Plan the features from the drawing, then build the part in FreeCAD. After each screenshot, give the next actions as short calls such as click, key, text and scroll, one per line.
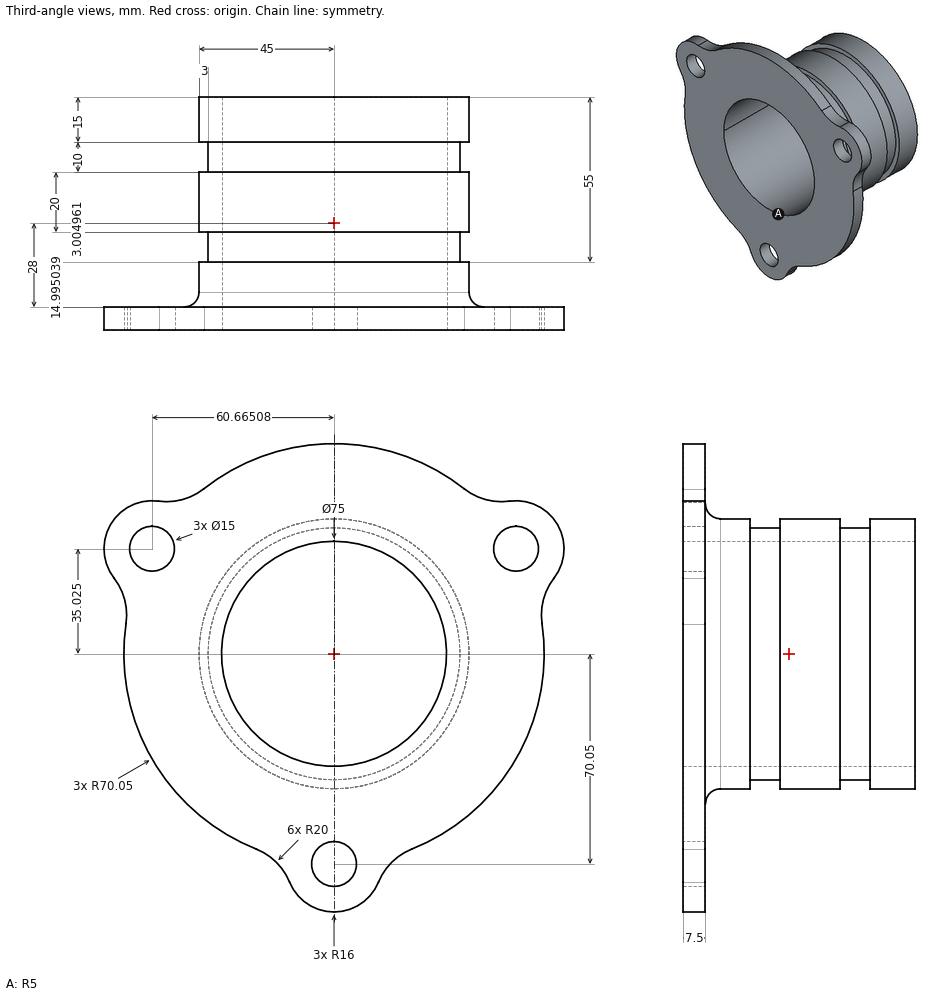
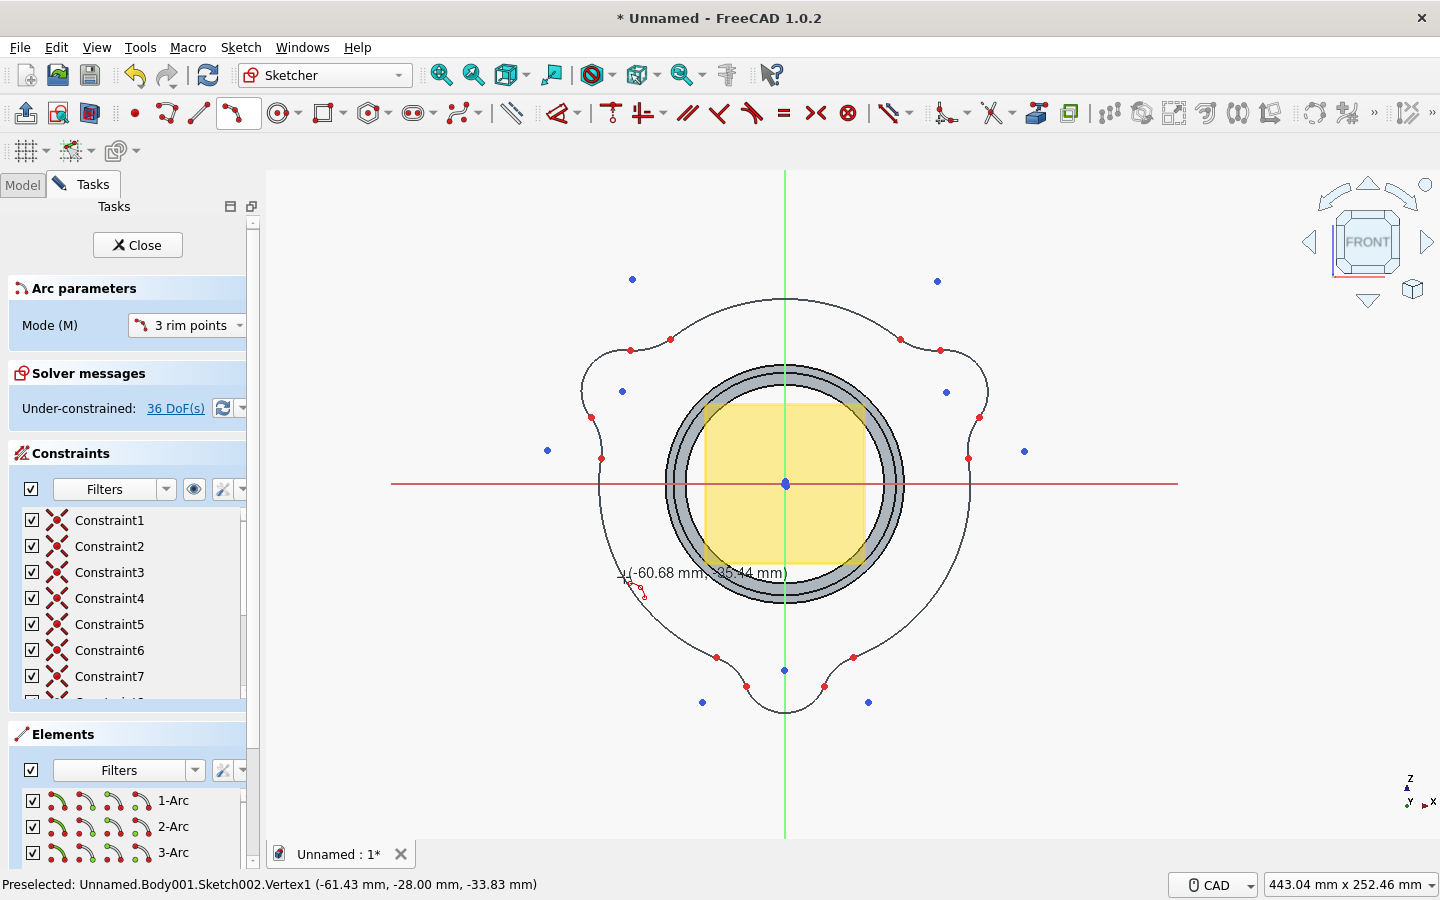
key(g)
key(c)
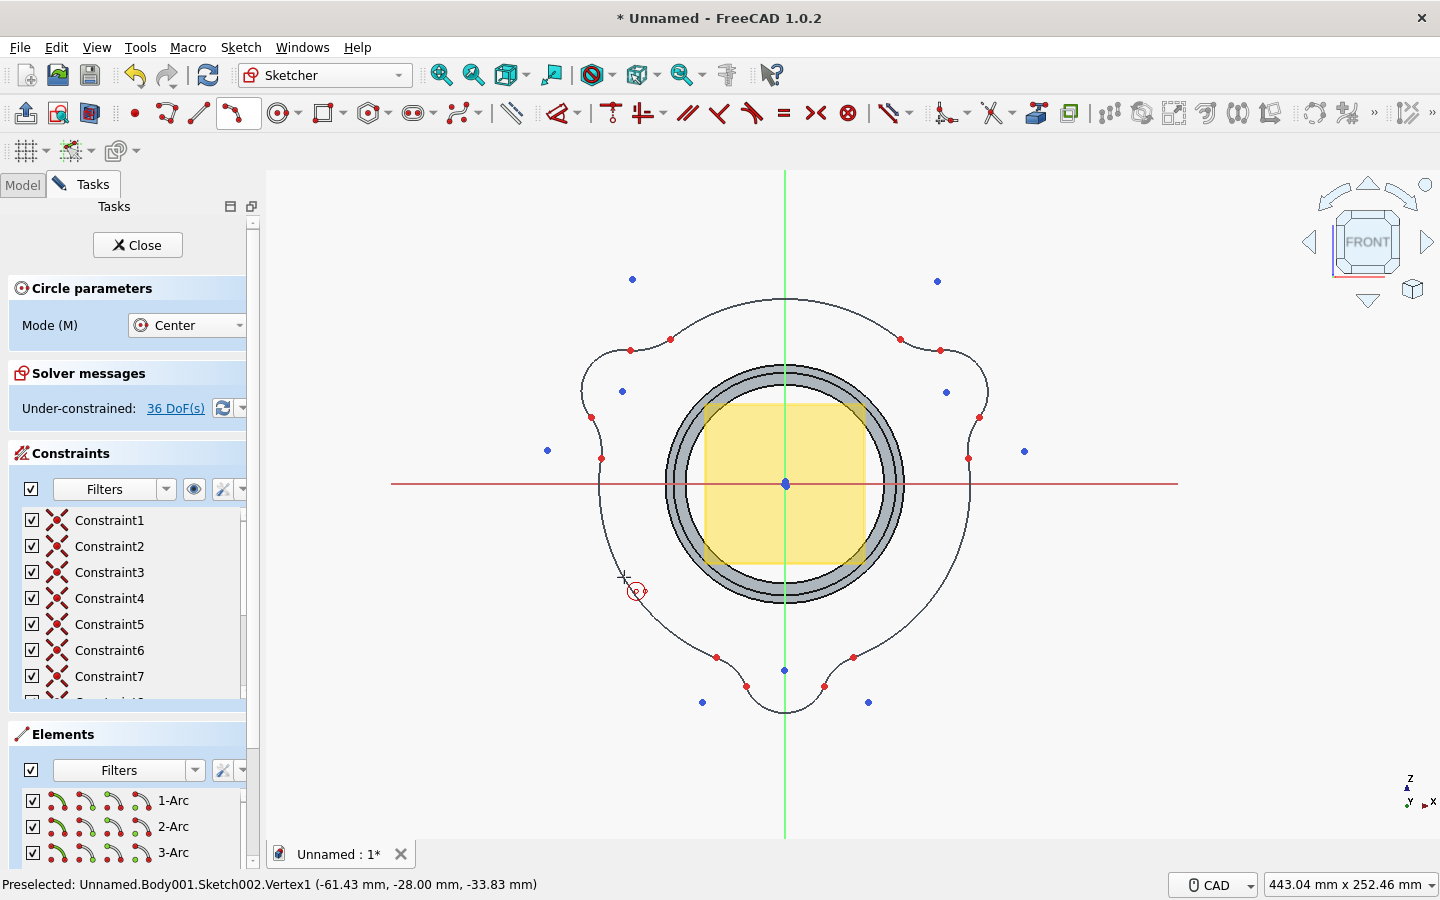
click(624, 391)
click(638, 377)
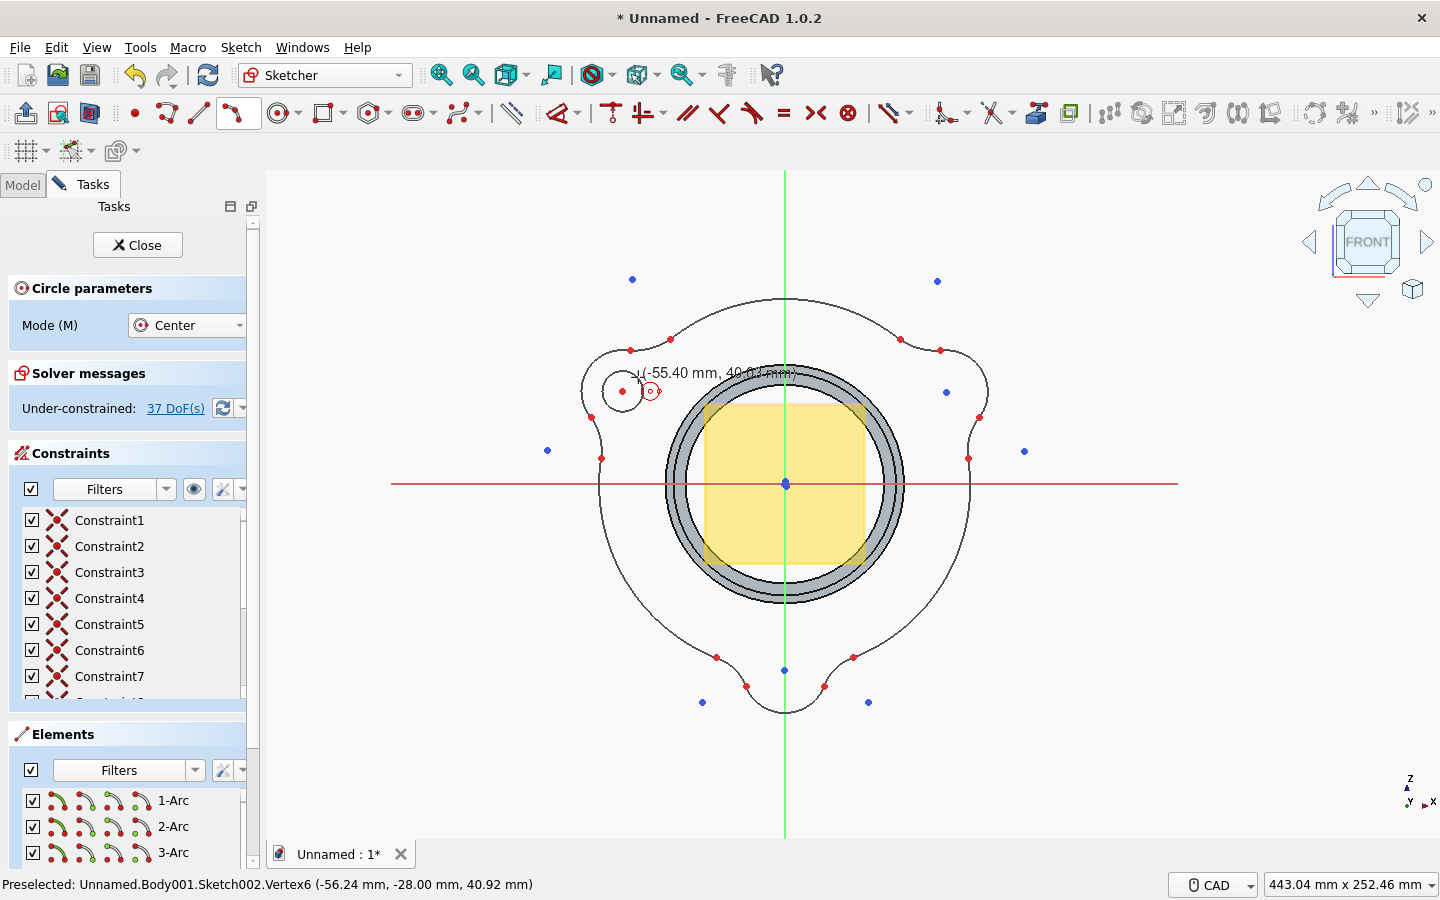
click(946, 391)
click(960, 377)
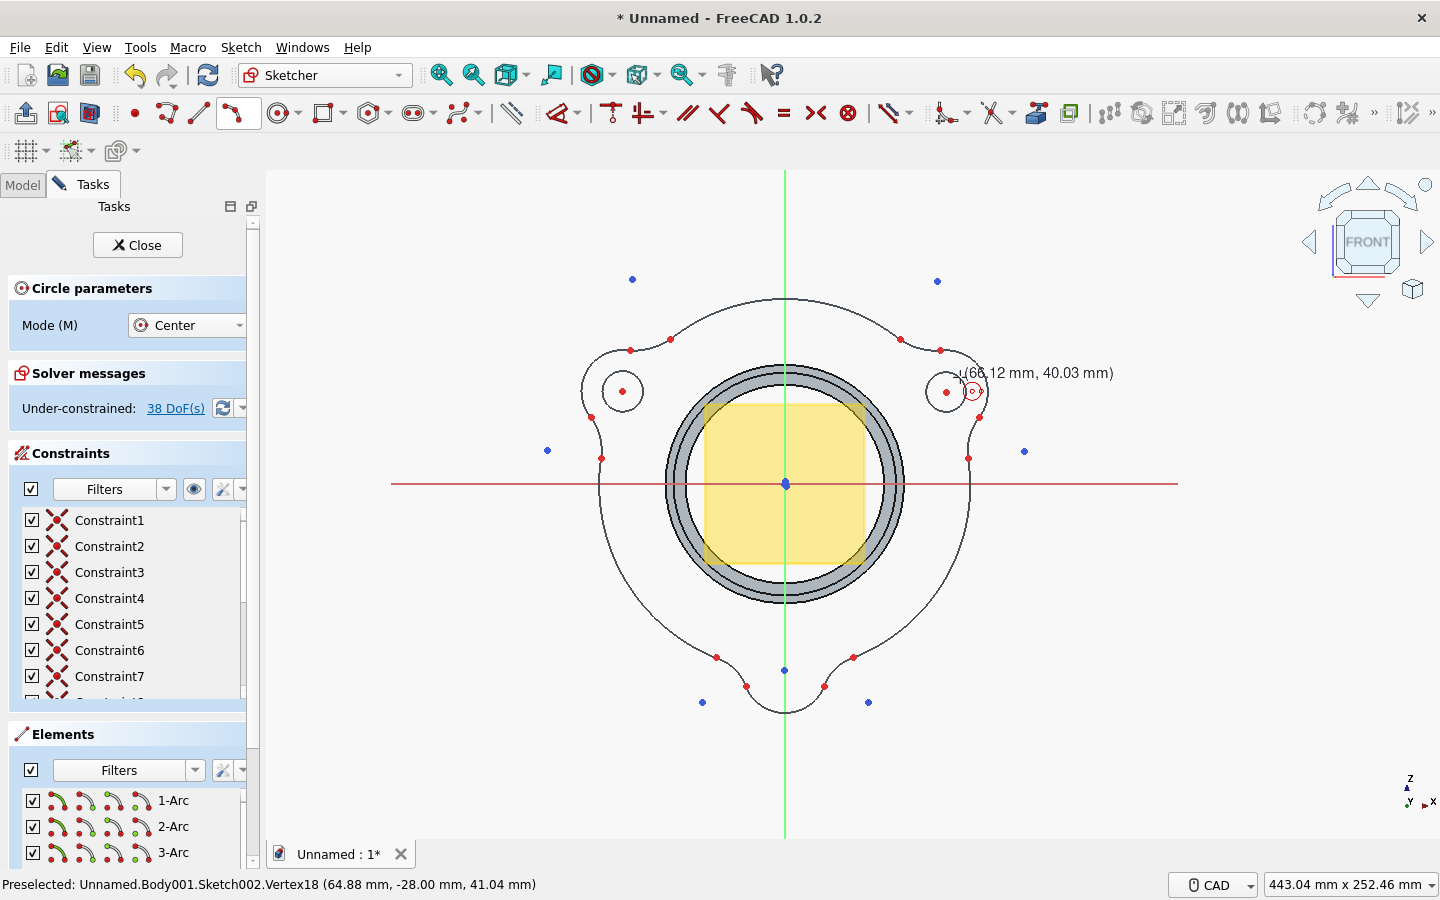
click(785, 670)
click(799, 656)
key(Escape)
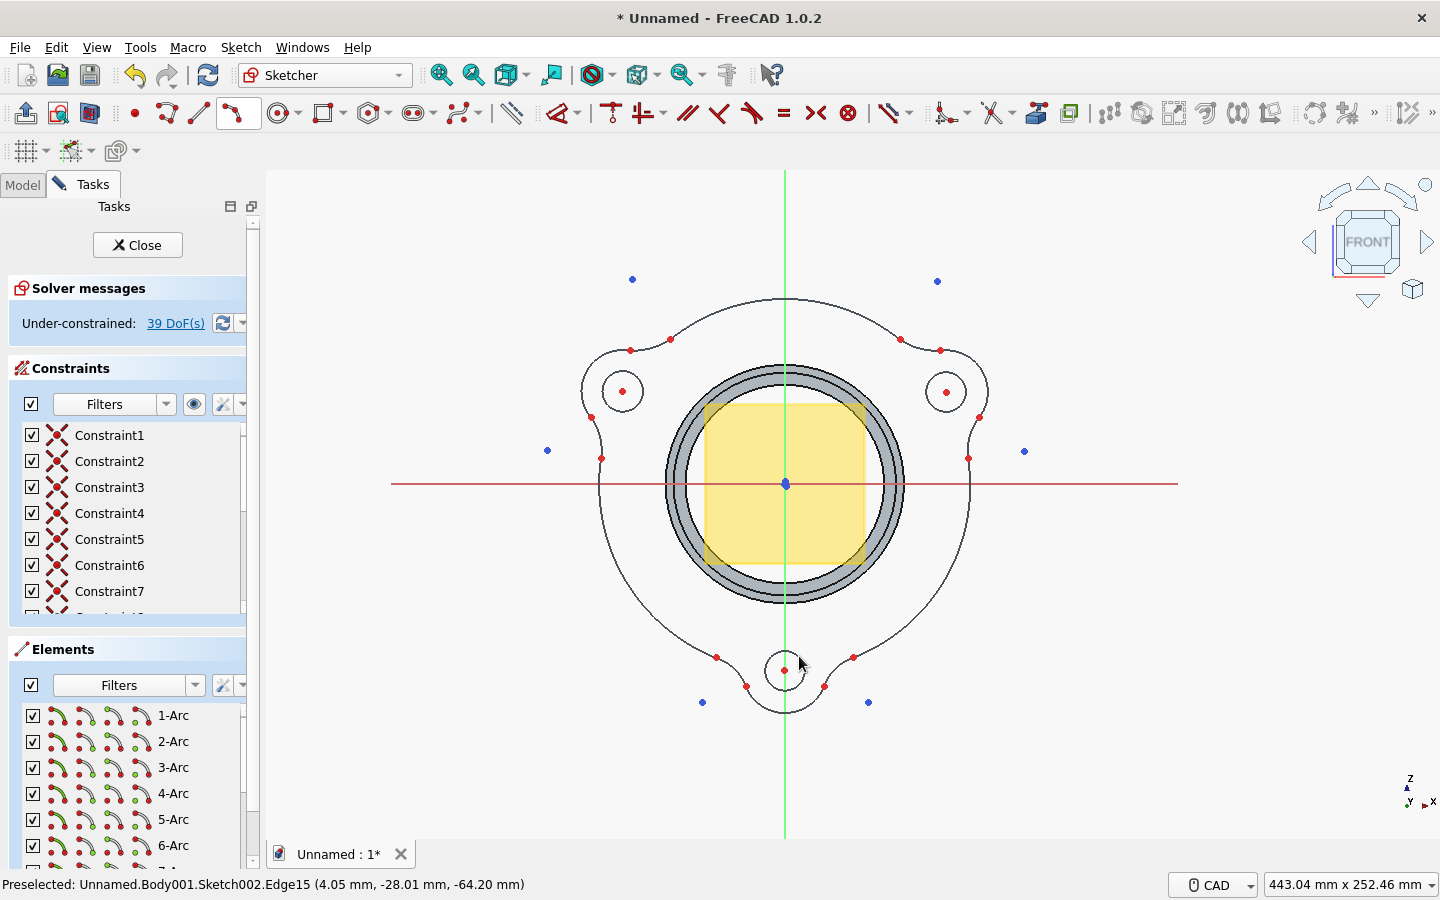
click(602, 446)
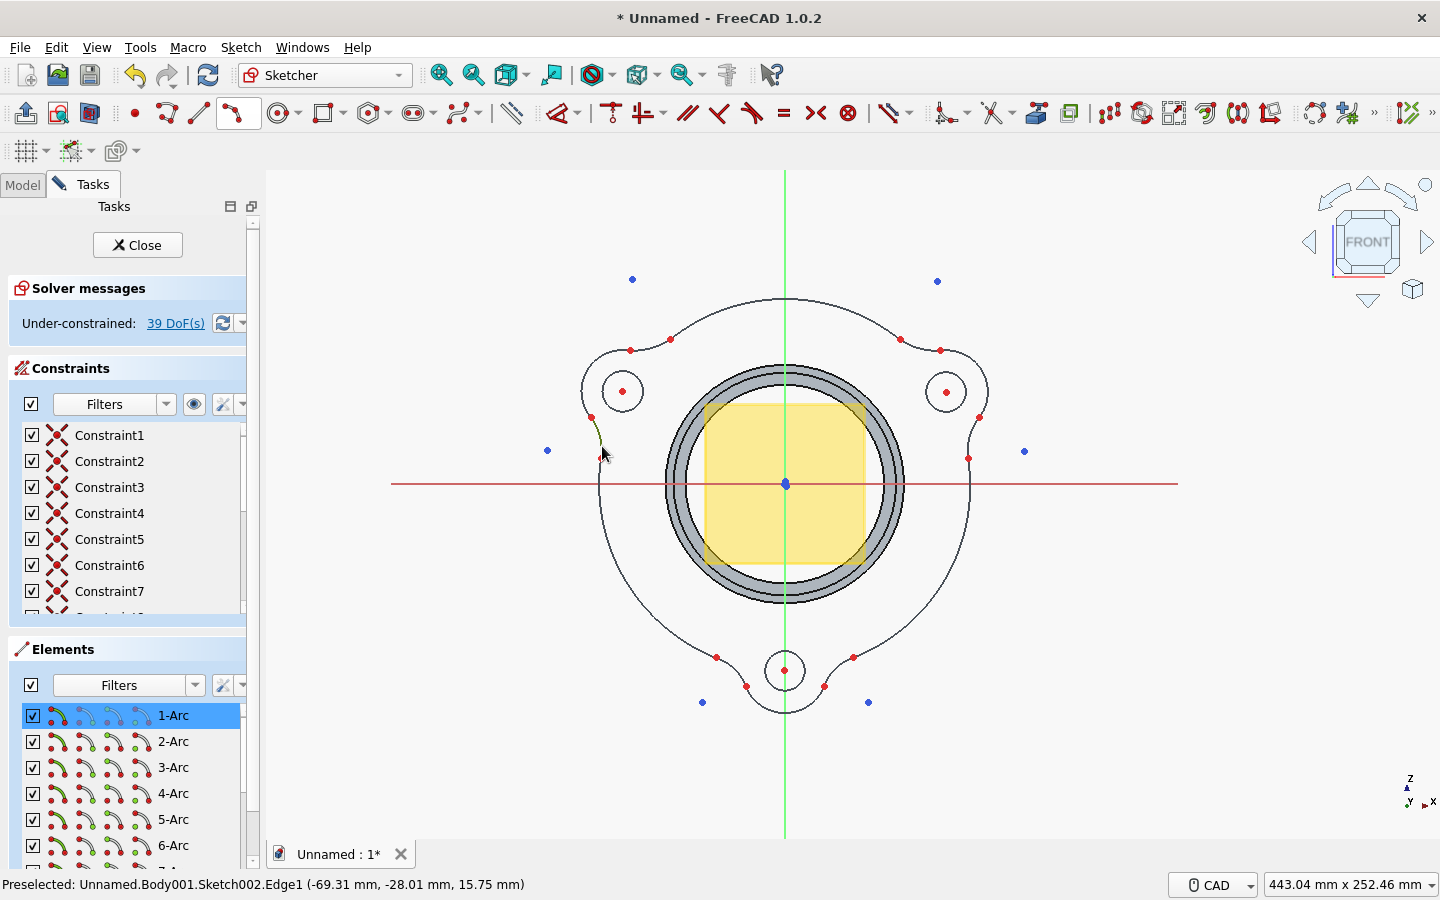
click(601, 356)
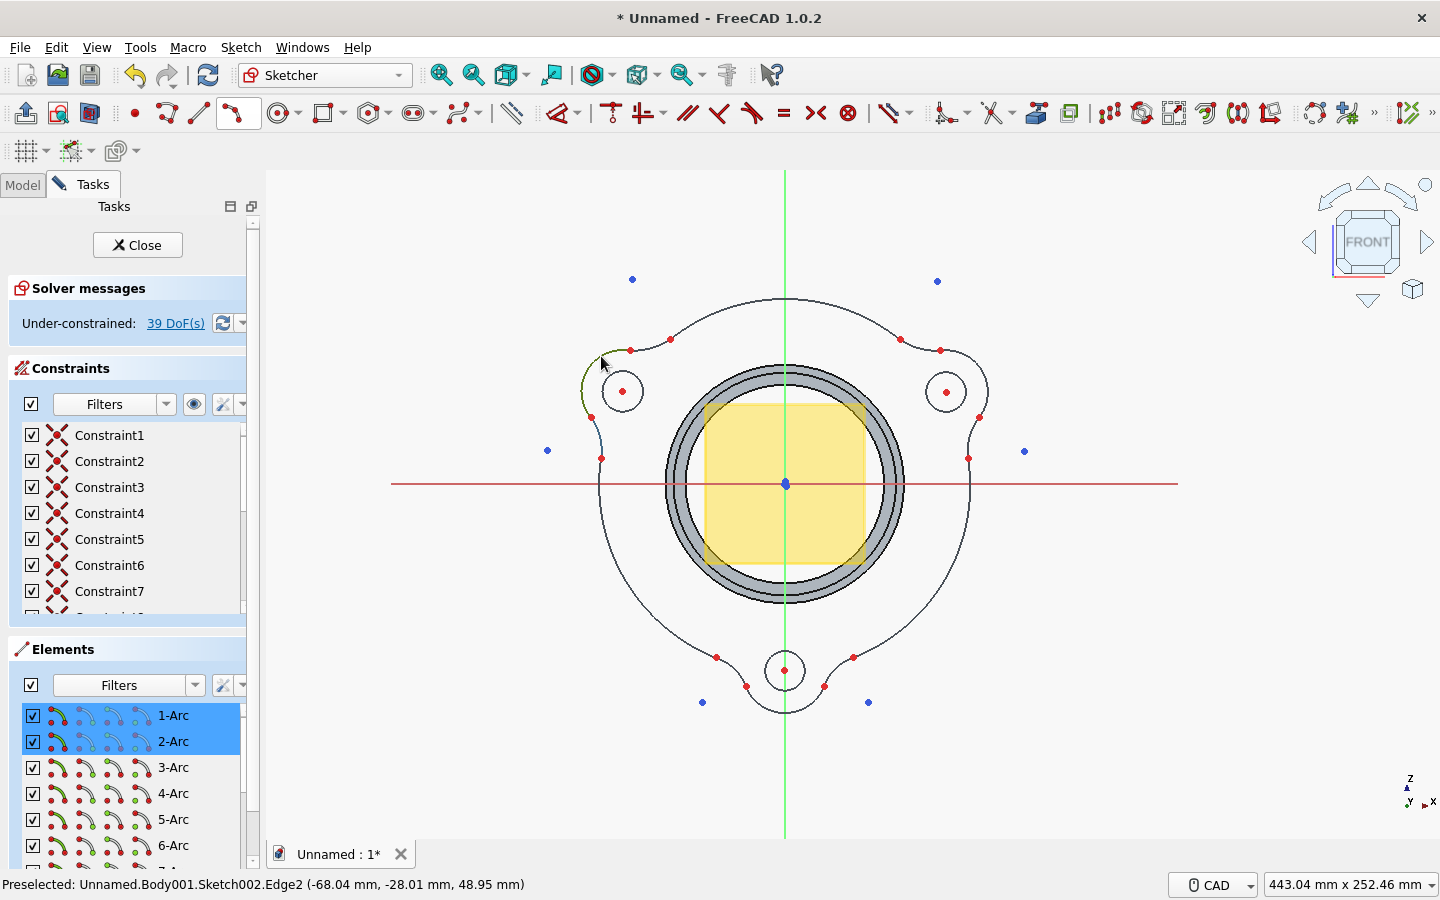
key(t)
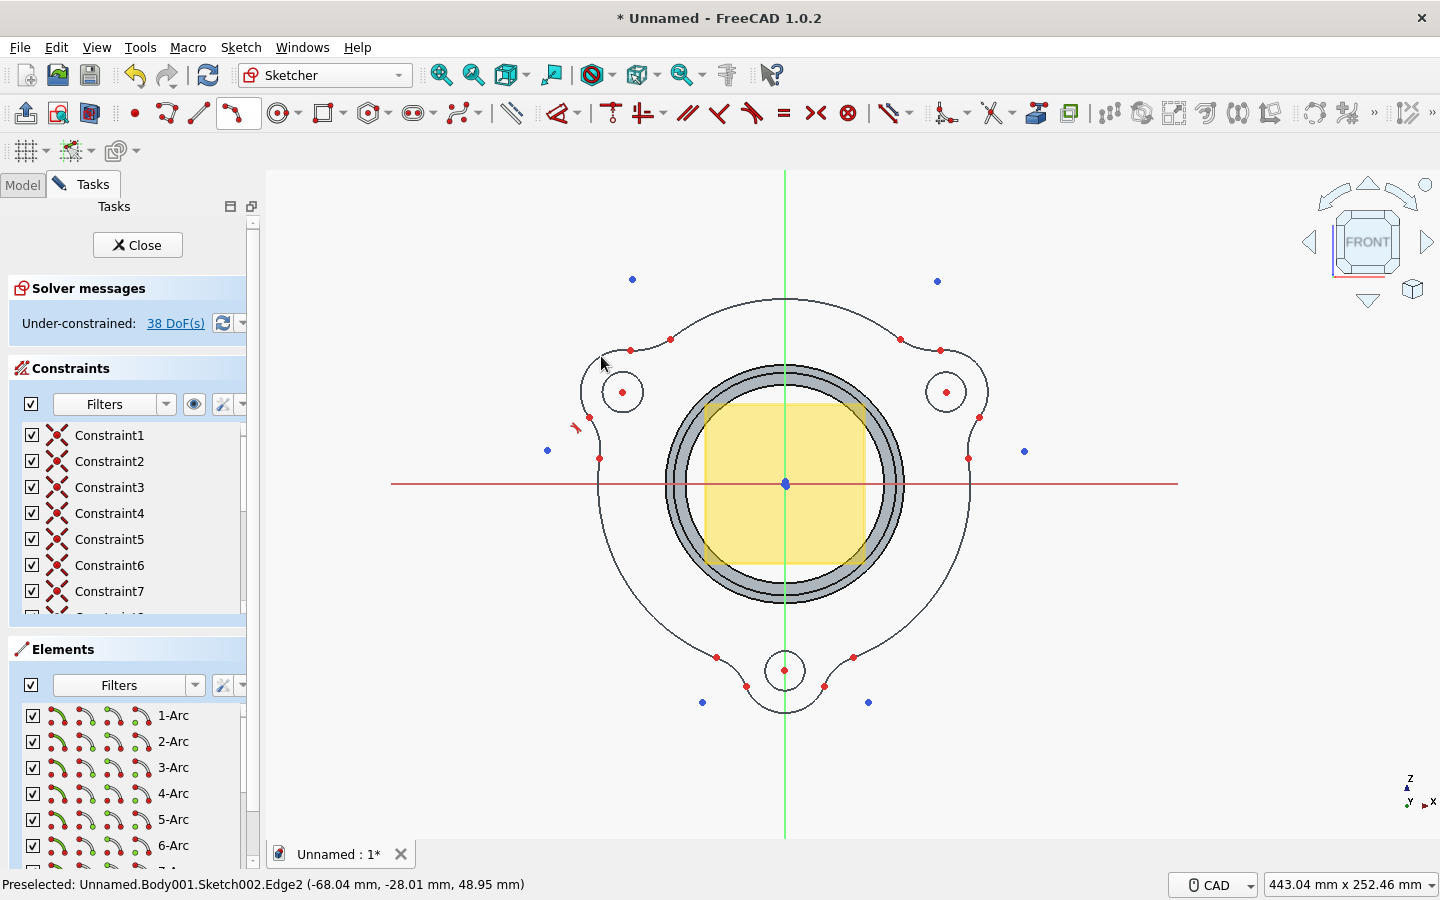
click(600, 446)